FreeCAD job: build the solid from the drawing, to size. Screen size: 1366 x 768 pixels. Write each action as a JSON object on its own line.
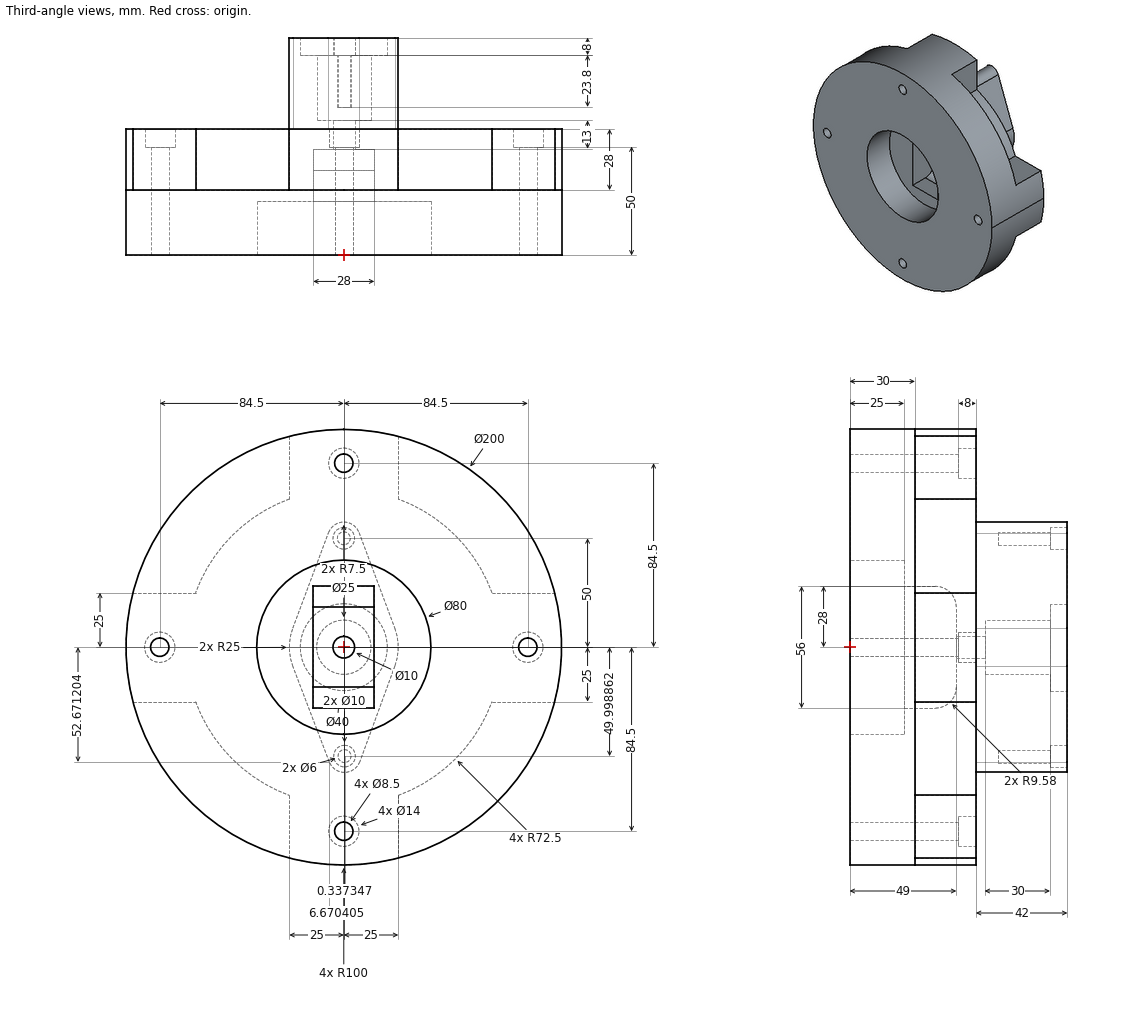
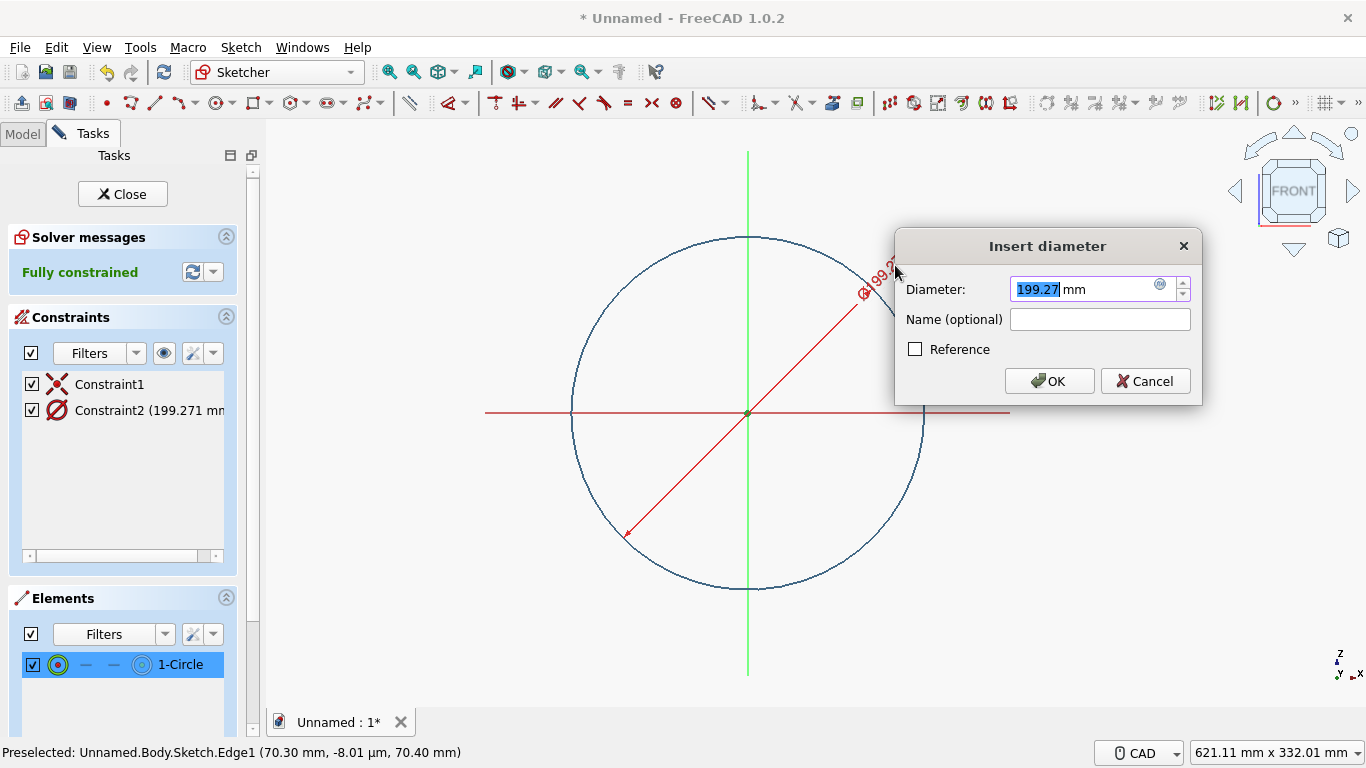
{"action": "type", "text": "200"}
{"action": "key", "text": "Return"}
{"action": "key", "text": "Escape"}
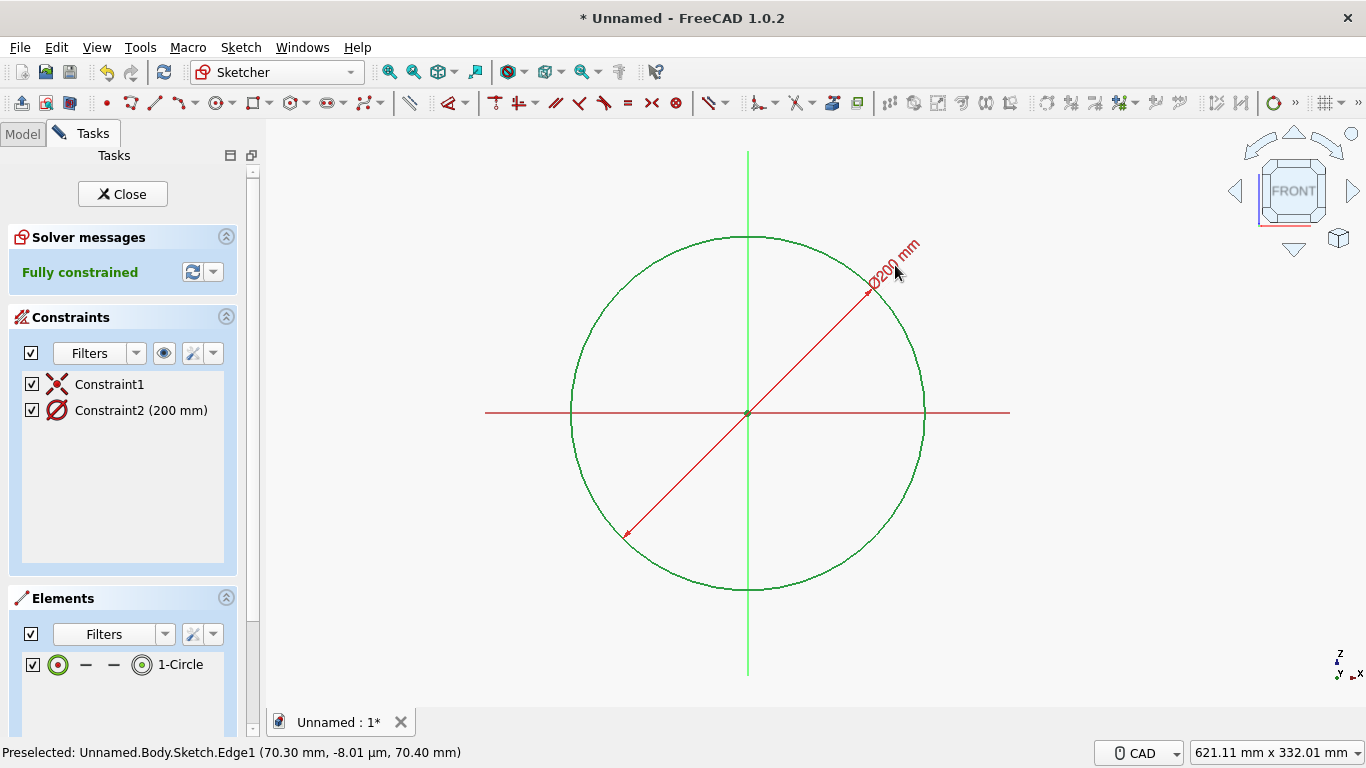
{"action": "left_click", "coordinate": [123, 194]}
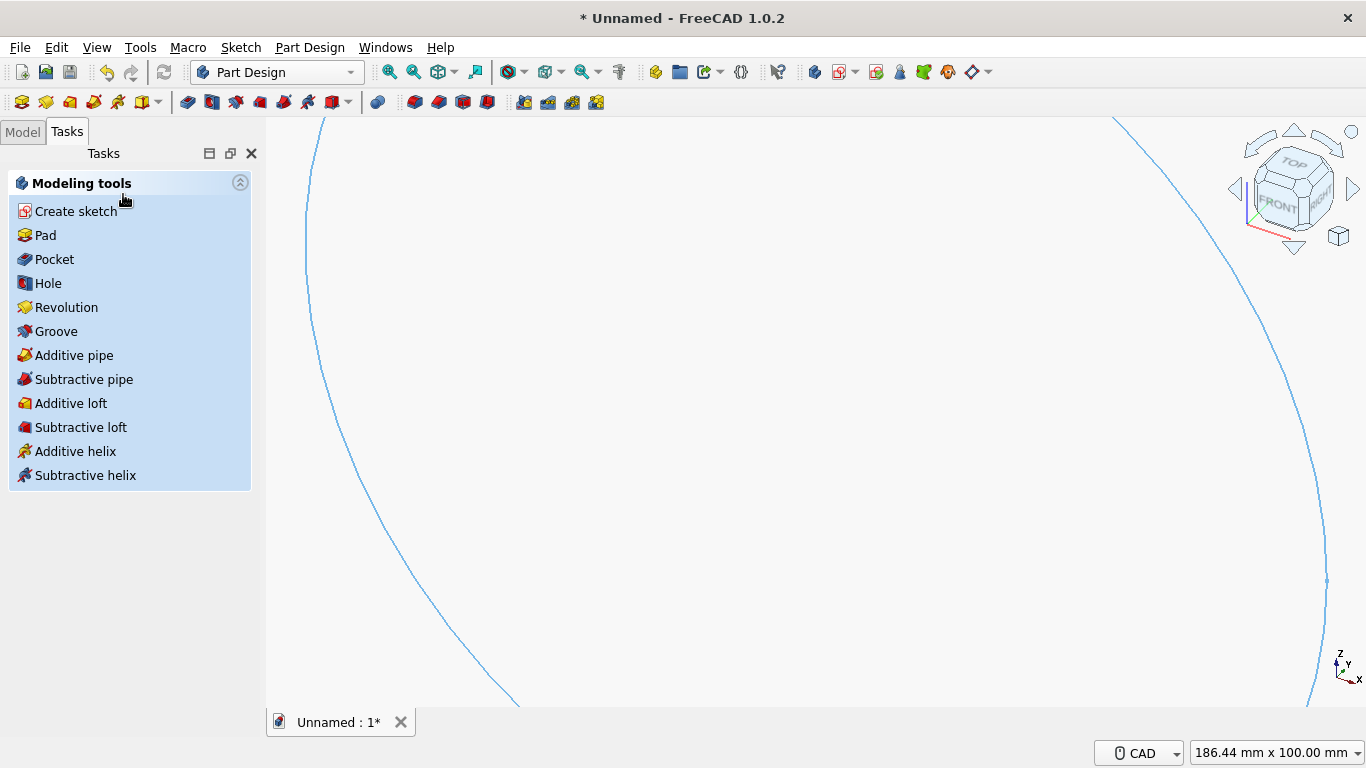
{"action": "left_click", "coordinate": [22, 102]}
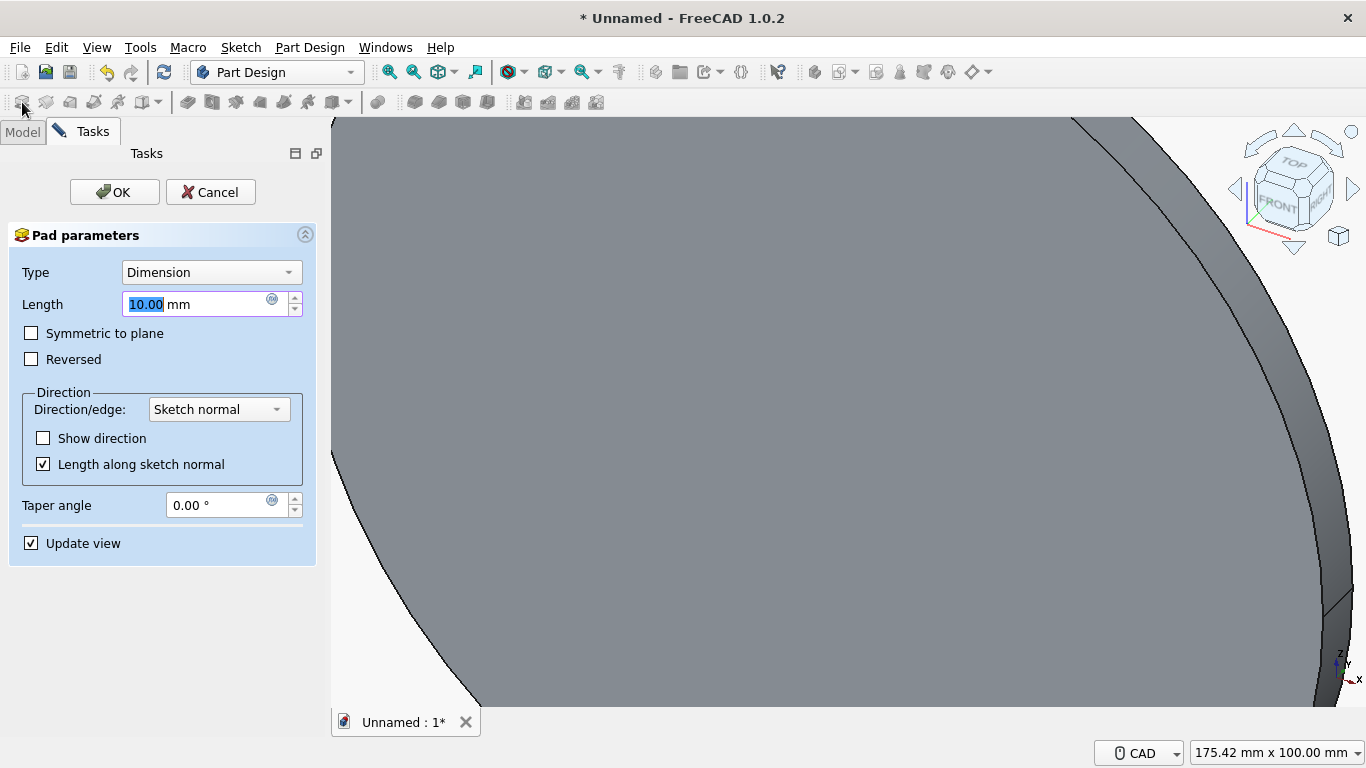
{"action": "type", "text": "30"}
{"action": "key", "text": "Tab"}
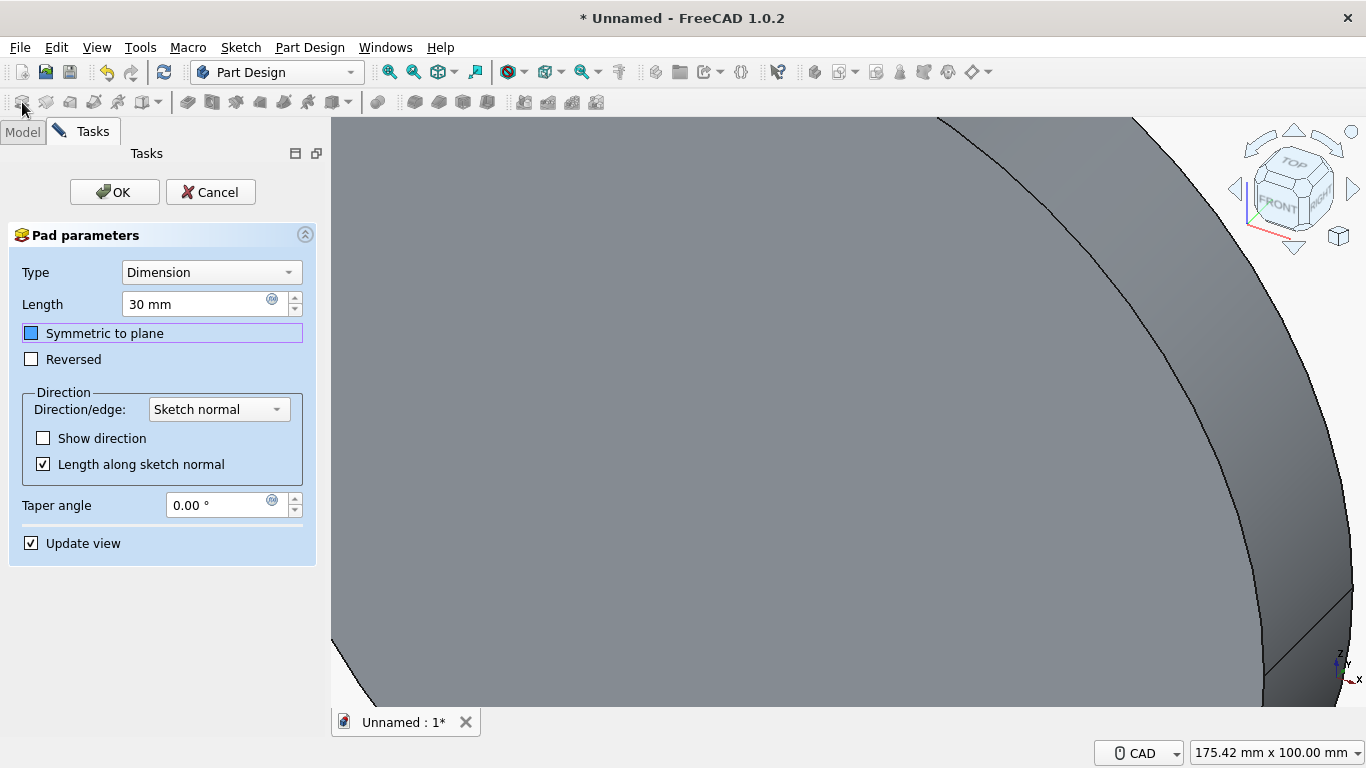
{"action": "left_click", "coordinate": [30, 359]}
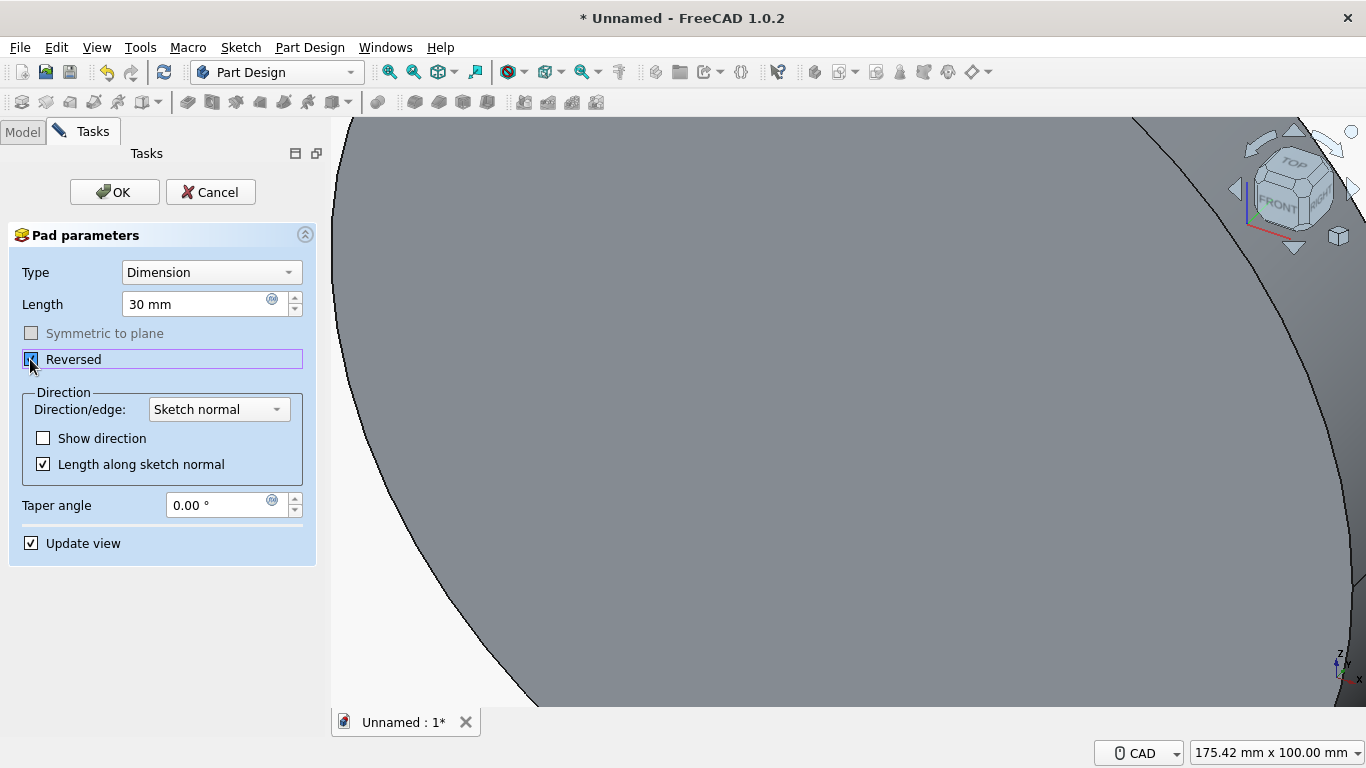
{"action": "left_click", "coordinate": [115, 192]}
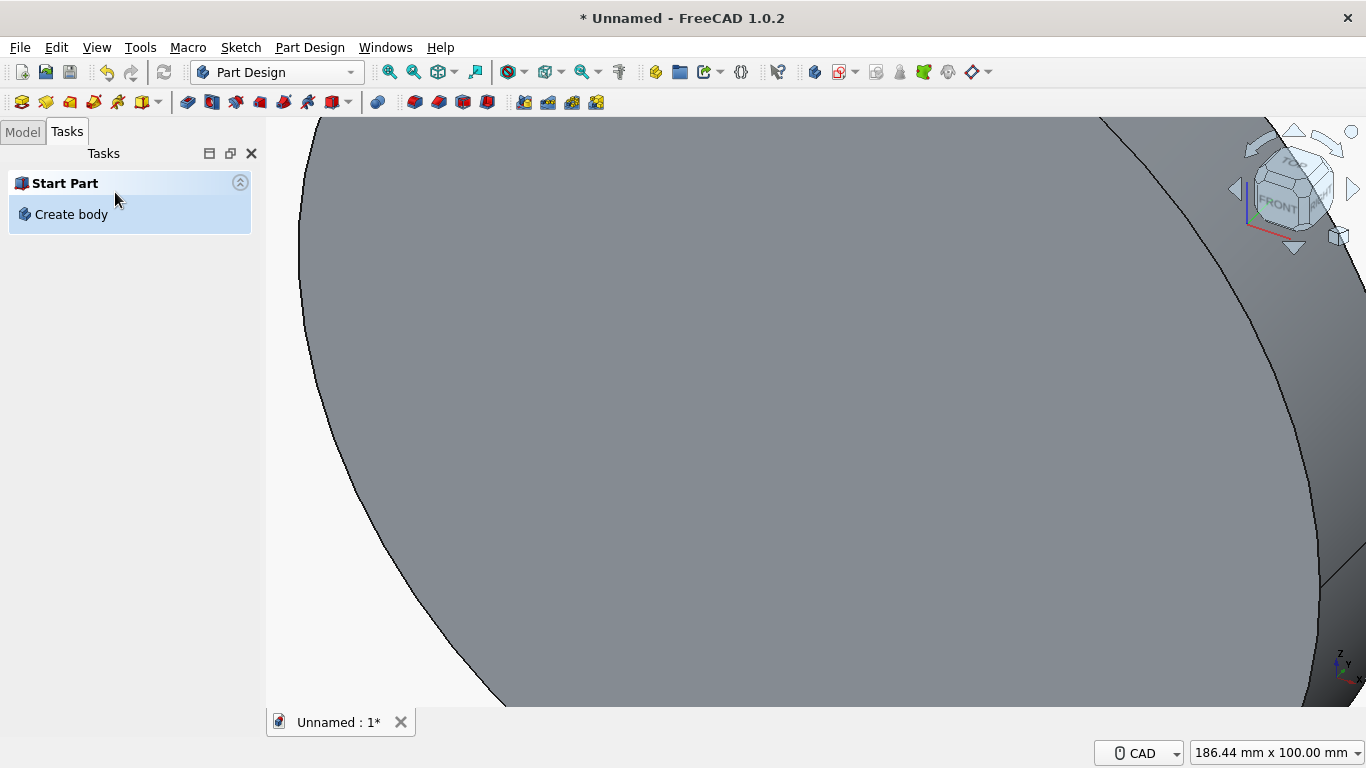
{"action": "key", "text": "v f"}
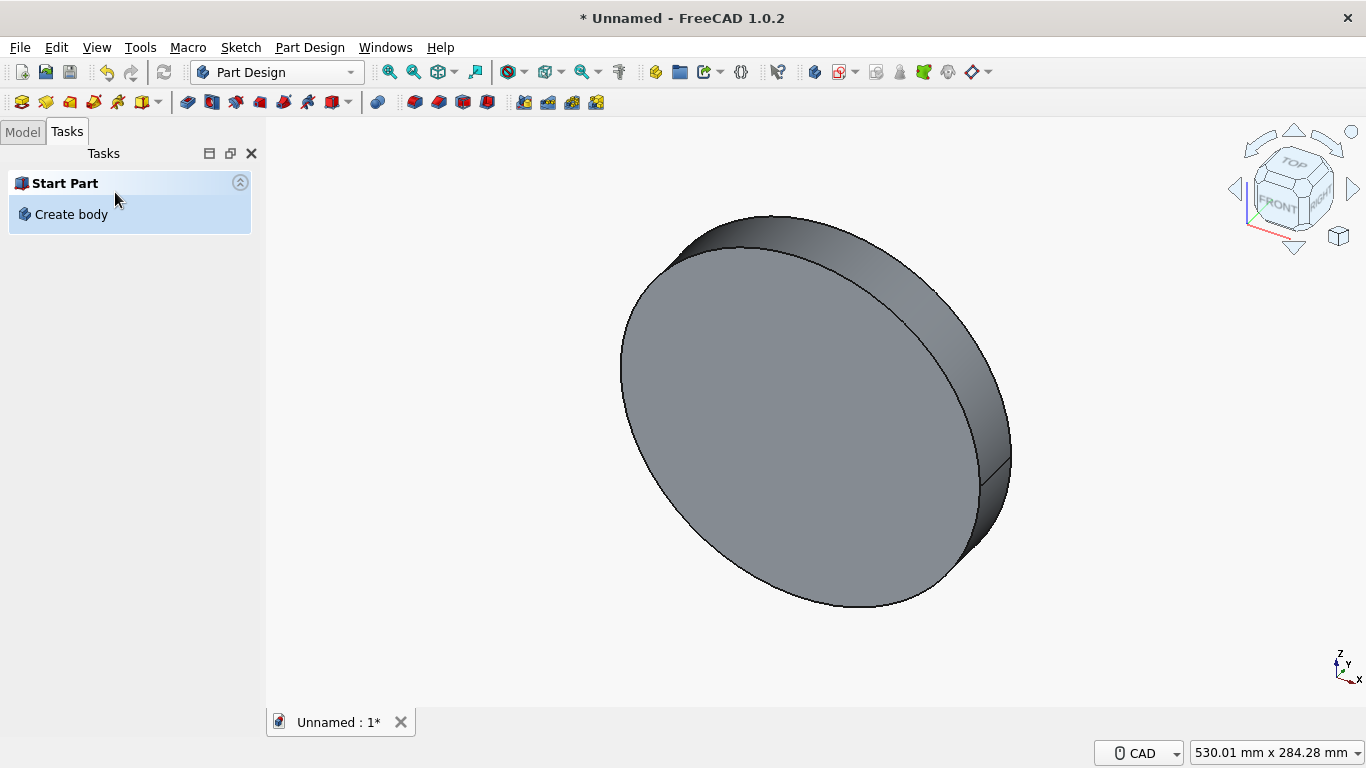
{"action": "key", "text": "4"}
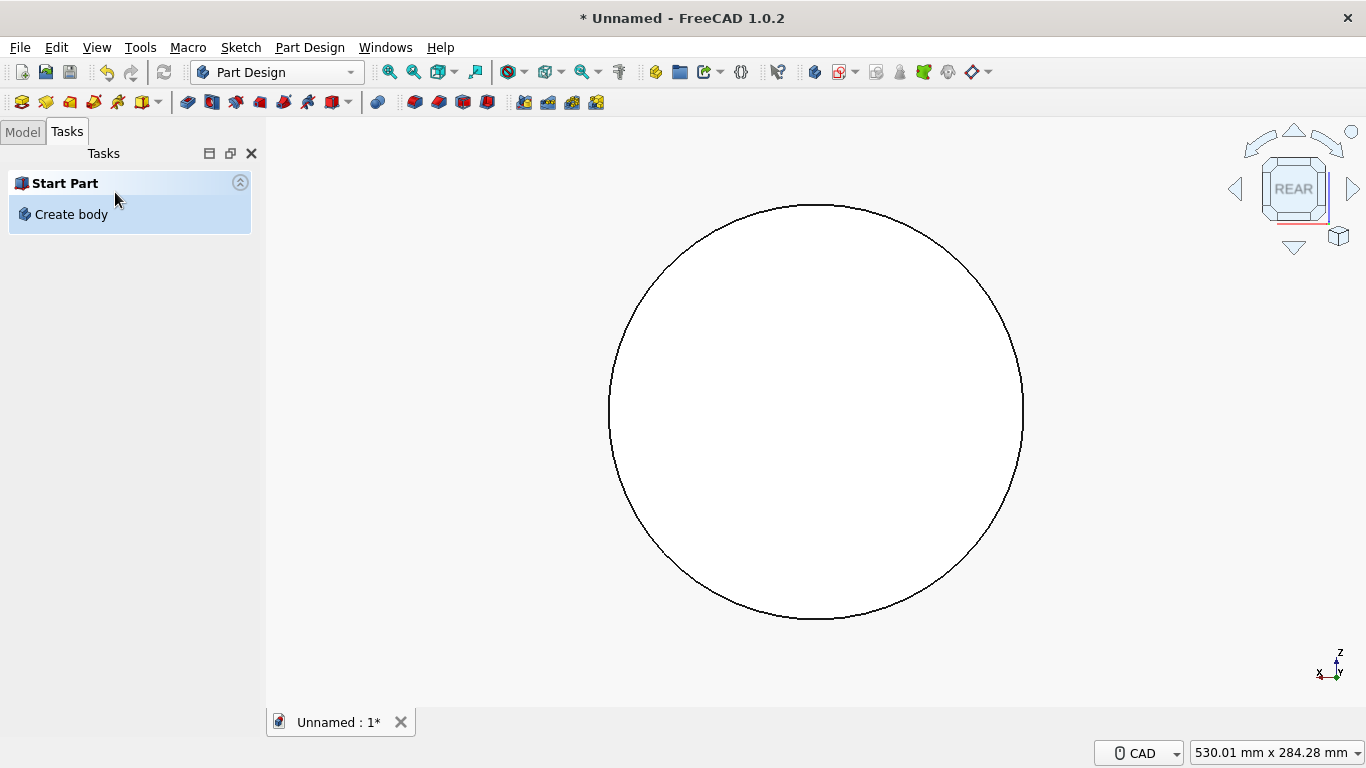
{"action": "left_click", "coordinate": [816, 411]}